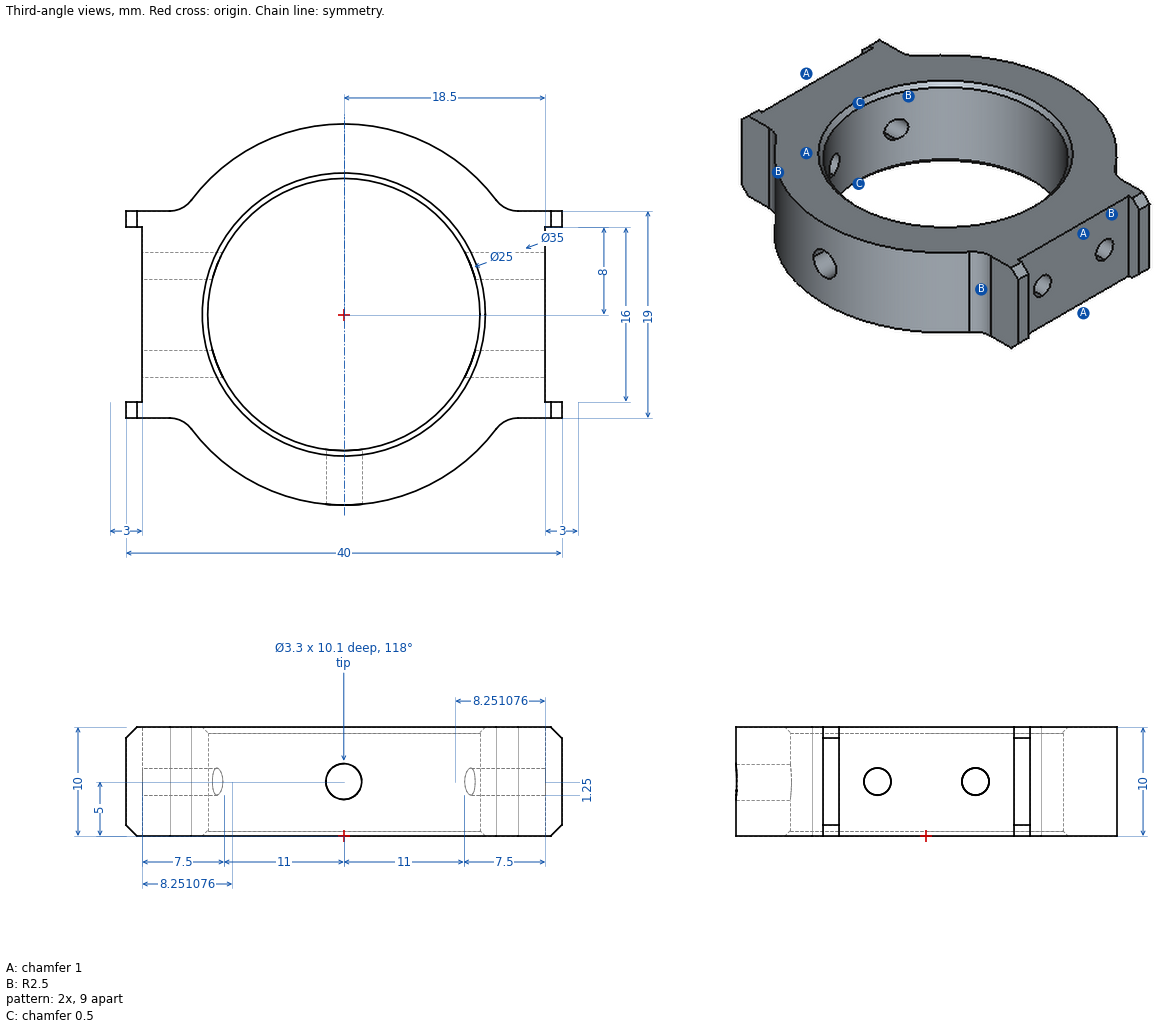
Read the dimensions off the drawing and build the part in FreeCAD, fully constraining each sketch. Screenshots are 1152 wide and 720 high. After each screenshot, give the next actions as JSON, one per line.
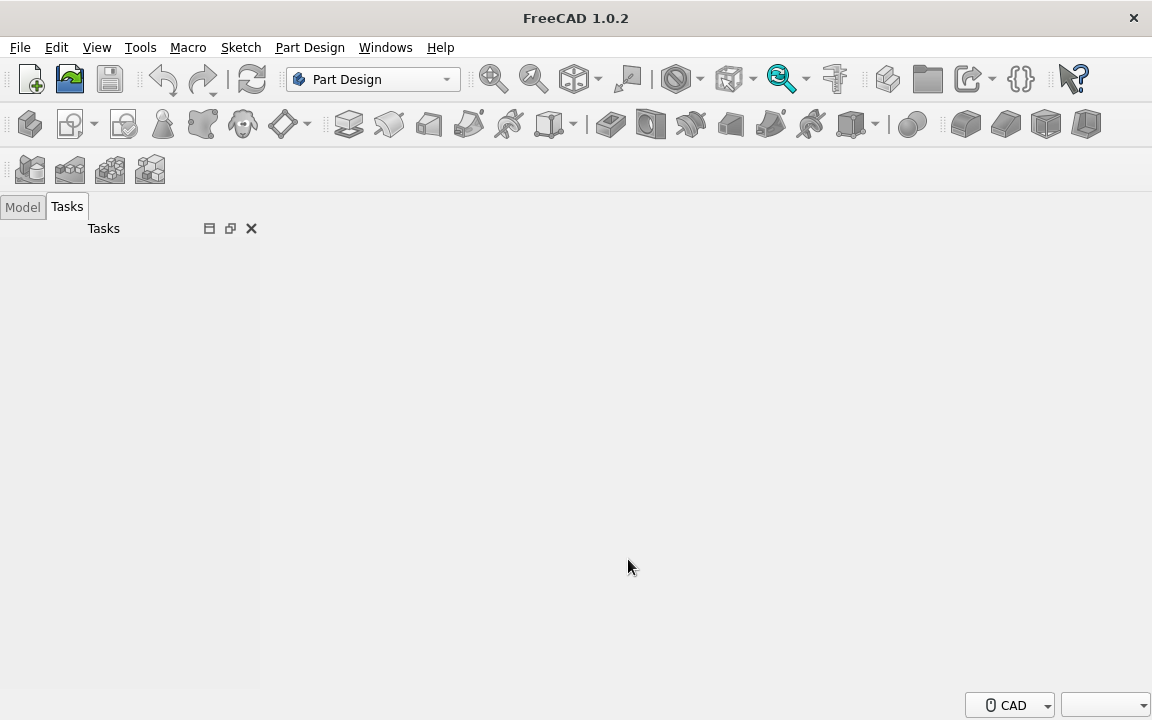
{"action": "key", "text": "ctrl+n"}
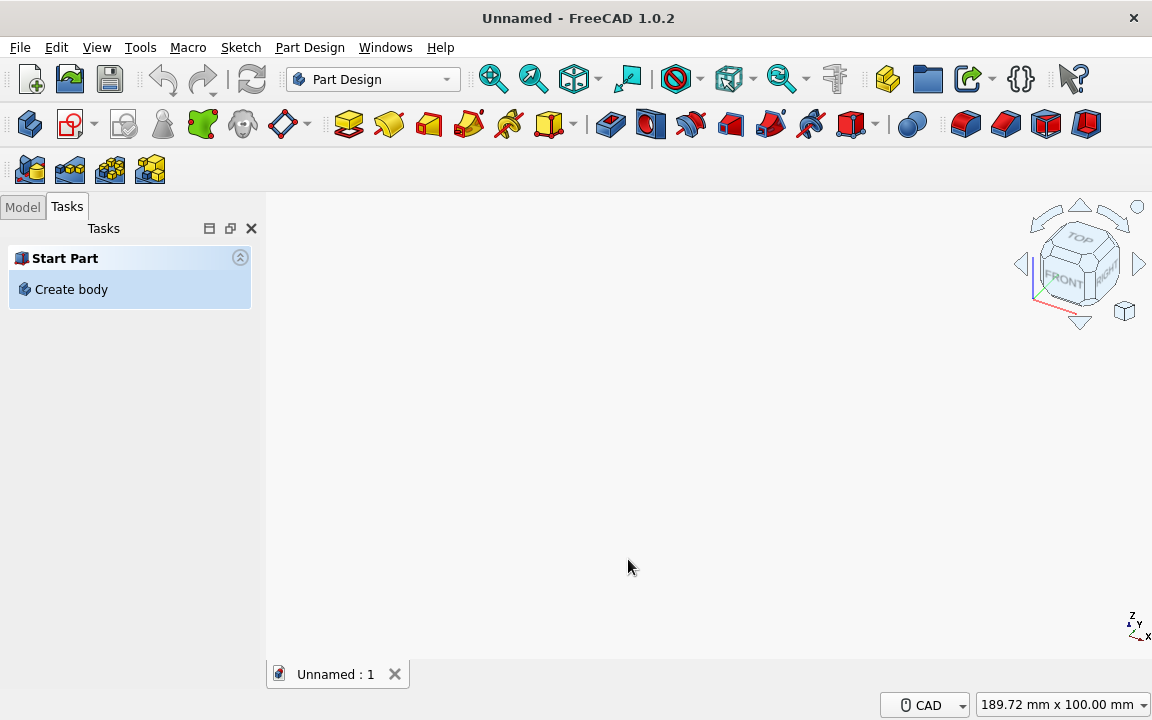
{"action": "left_click", "coordinate": [70, 124]}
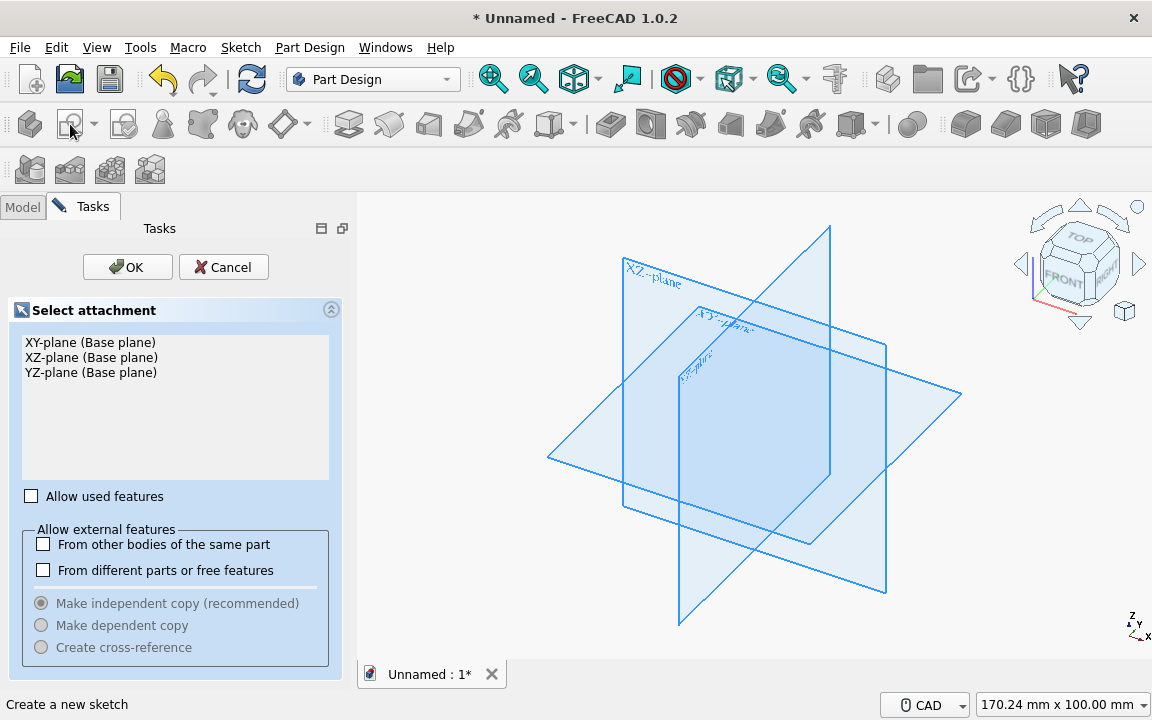
{"action": "left_click", "coordinate": [82, 342]}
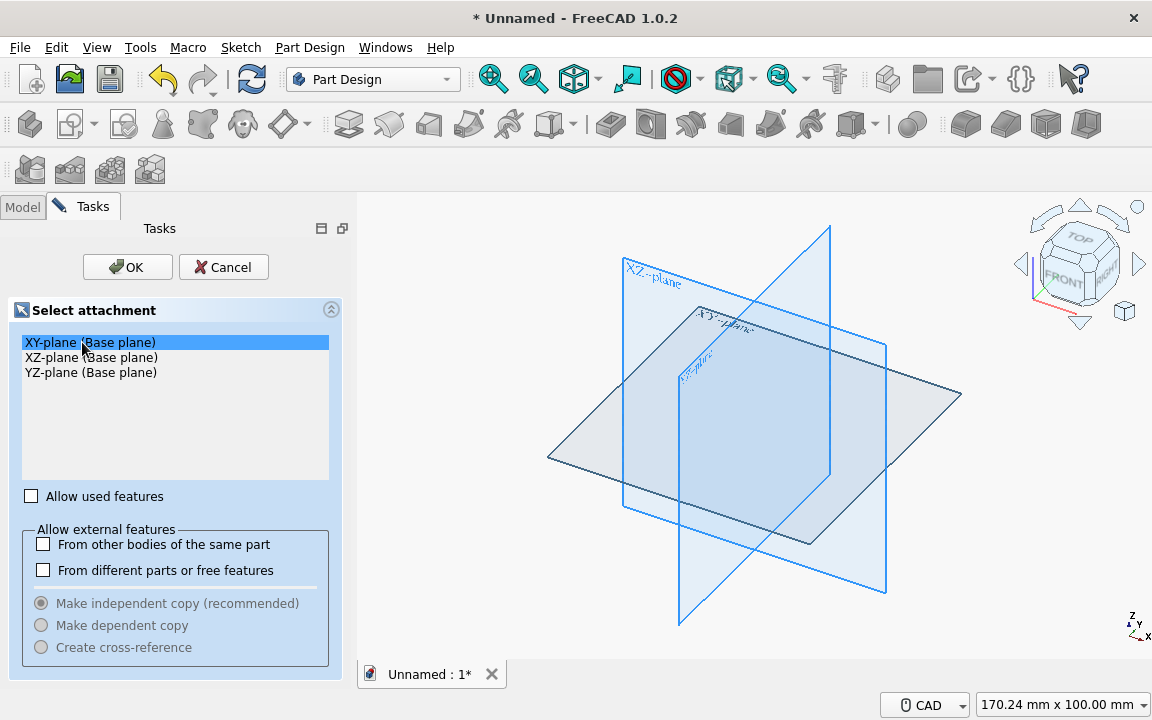
{"action": "left_click", "coordinate": [128, 267]}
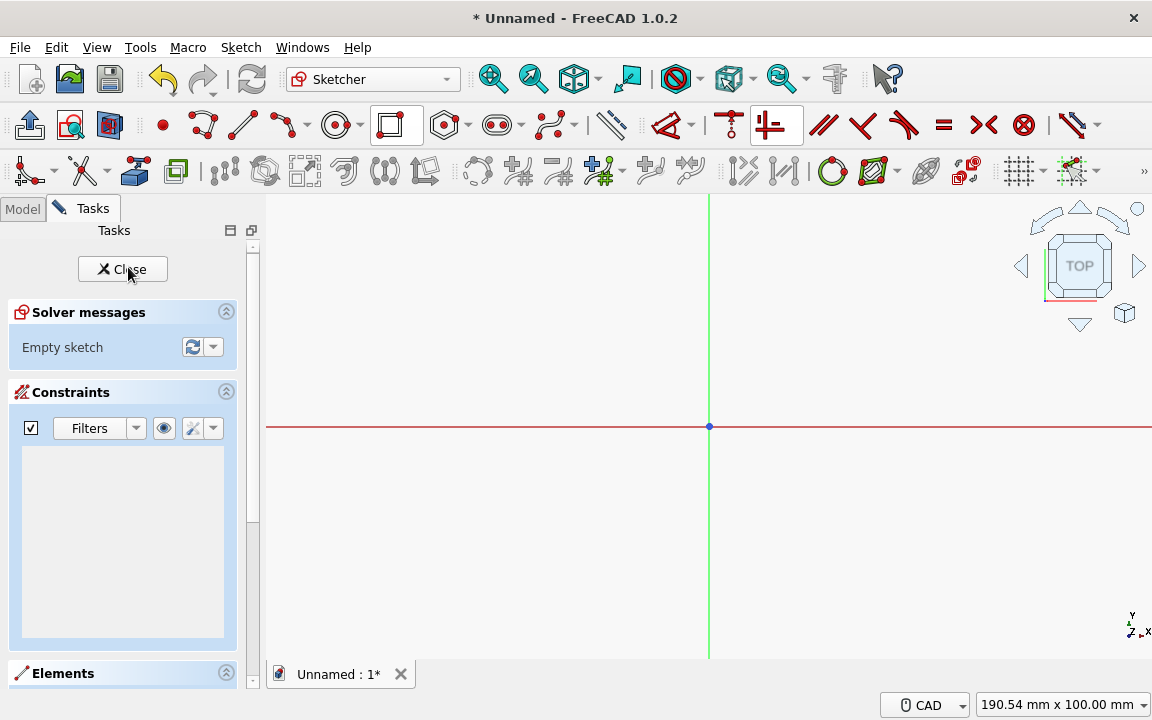
{"action": "scroll", "coordinate": [792, 426], "scroll_direction": "up", "scroll_amount": 3}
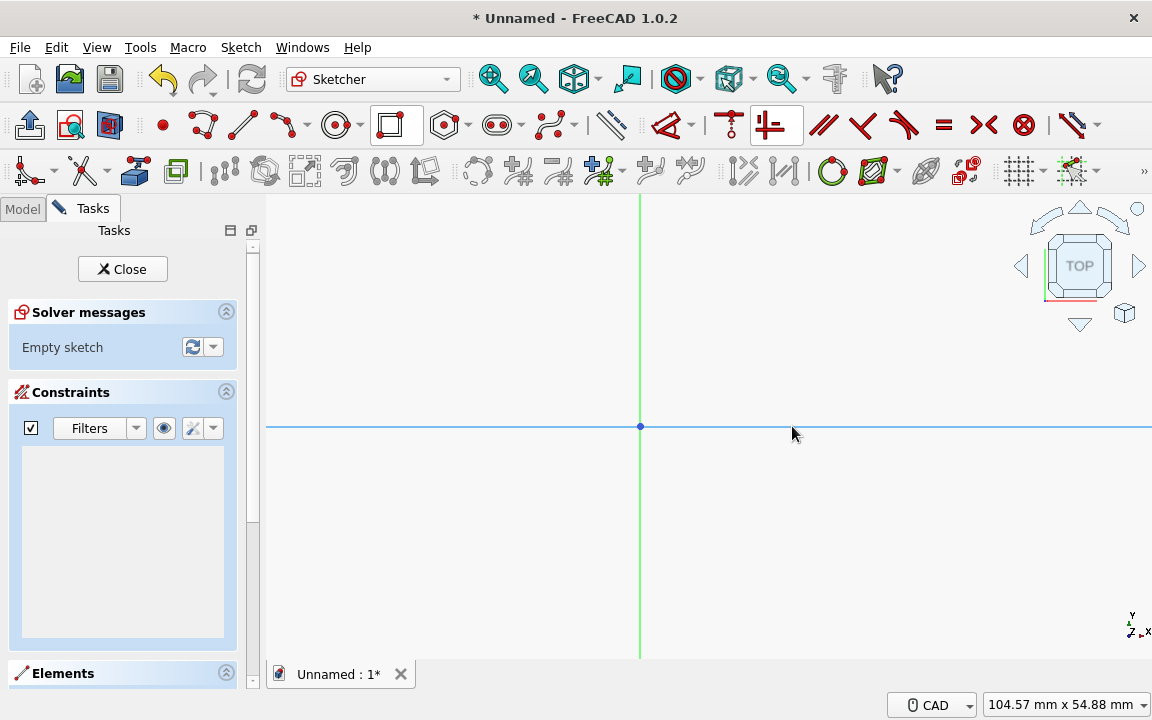
{"action": "left_click", "coordinate": [336, 126]}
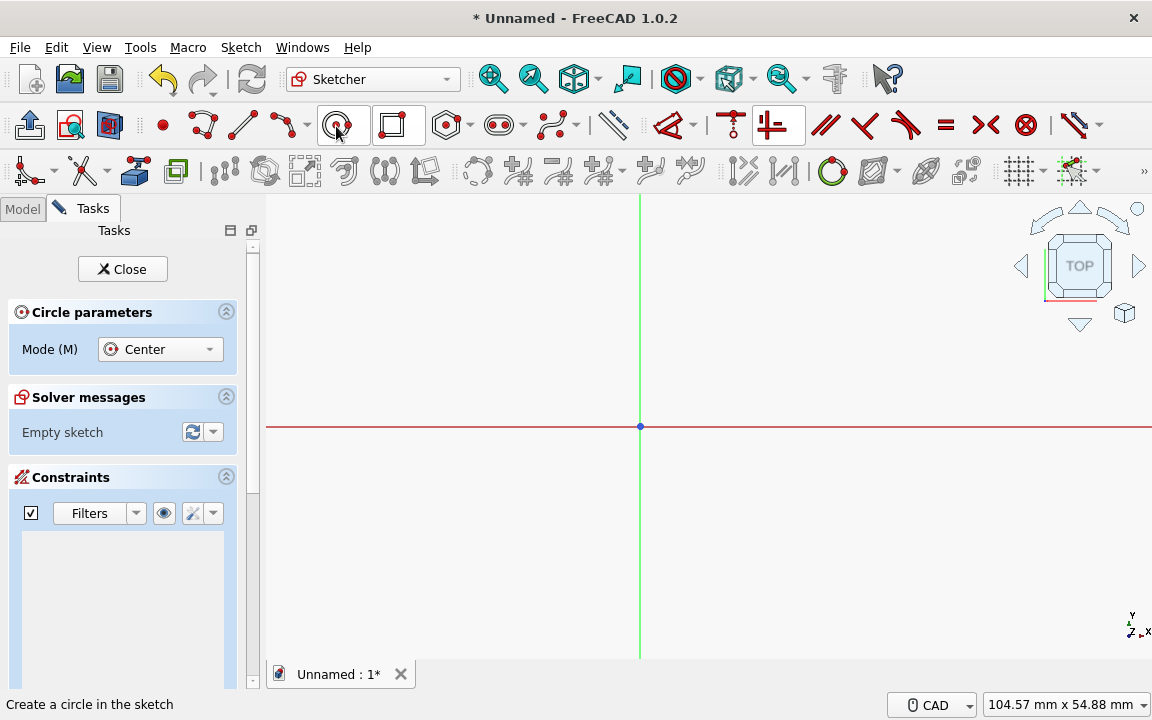
{"action": "left_click", "coordinate": [640, 426]}
{"action": "mouse_move", "coordinate": [745, 322]}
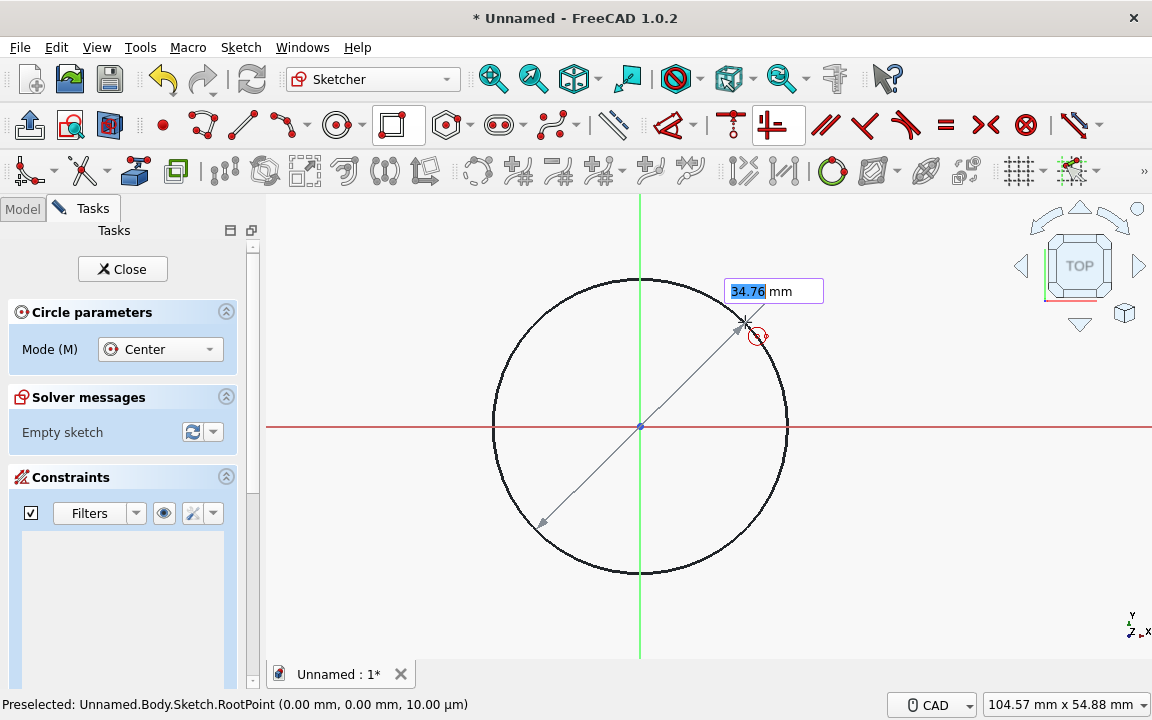
{"action": "type", "text": "35"}
{"action": "key", "text": "Return"}
{"action": "key", "text": "Escape"}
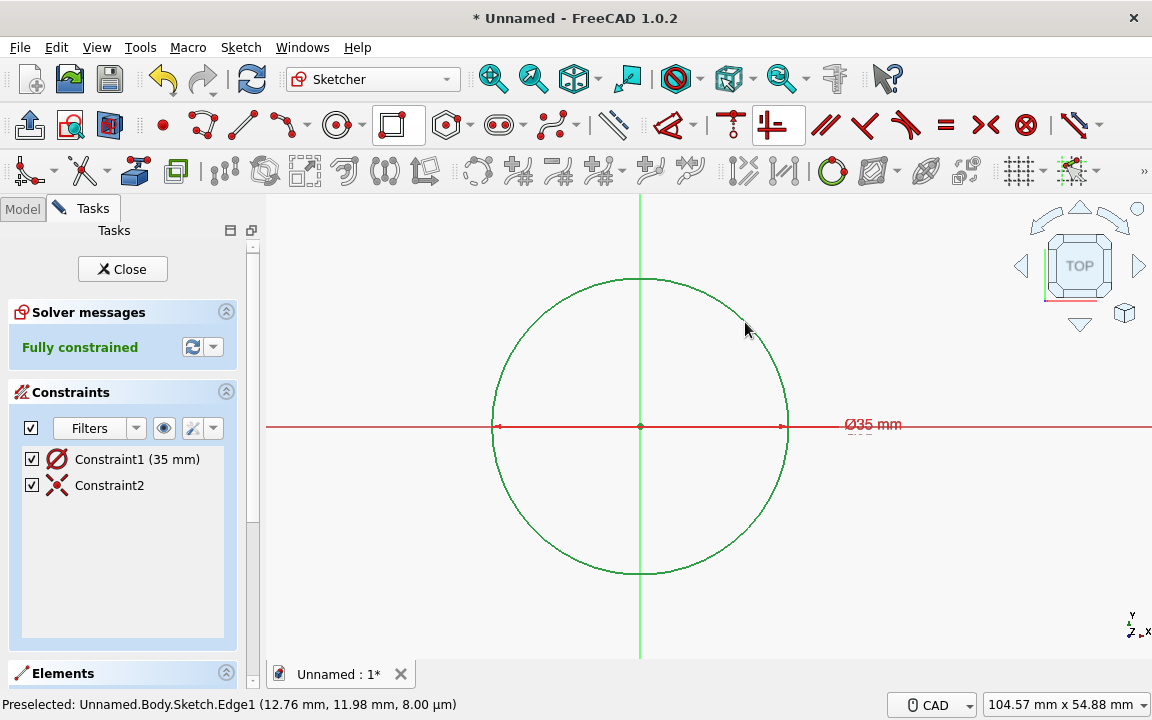
{"action": "left_click", "coordinate": [123, 269]}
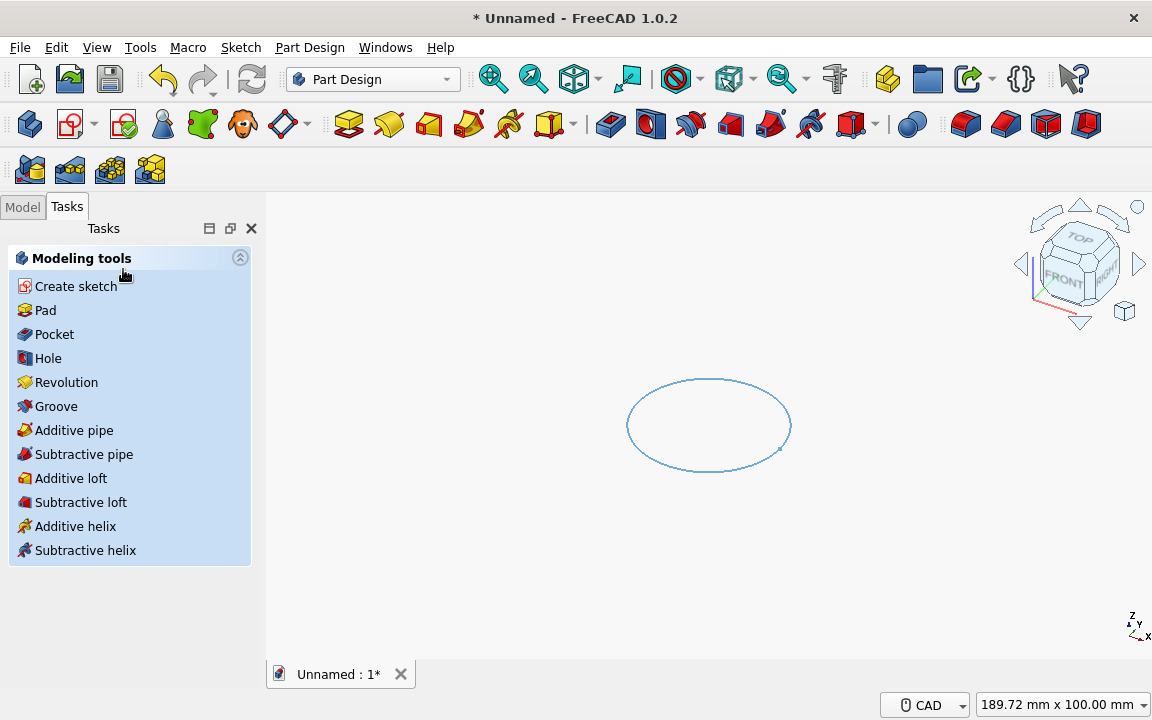
{"action": "left_click", "coordinate": [350, 124]}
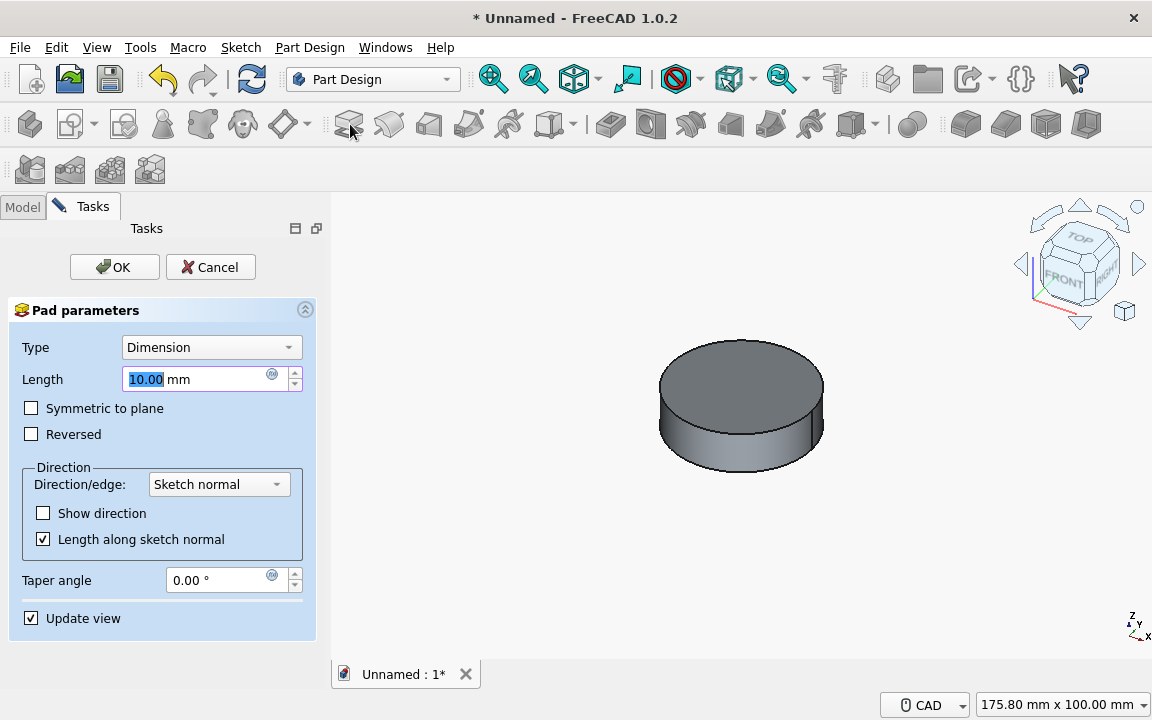
{"action": "type", "text": "10"}
{"action": "key", "text": "Tab"}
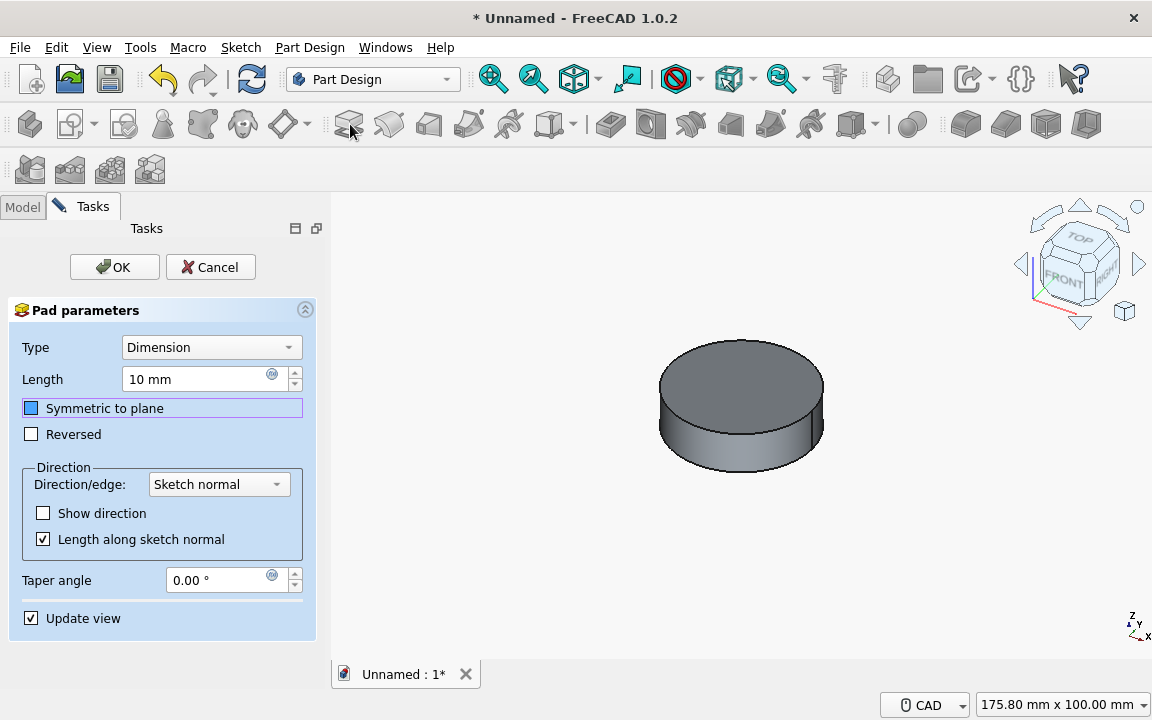
{"action": "left_click", "coordinate": [115, 267]}